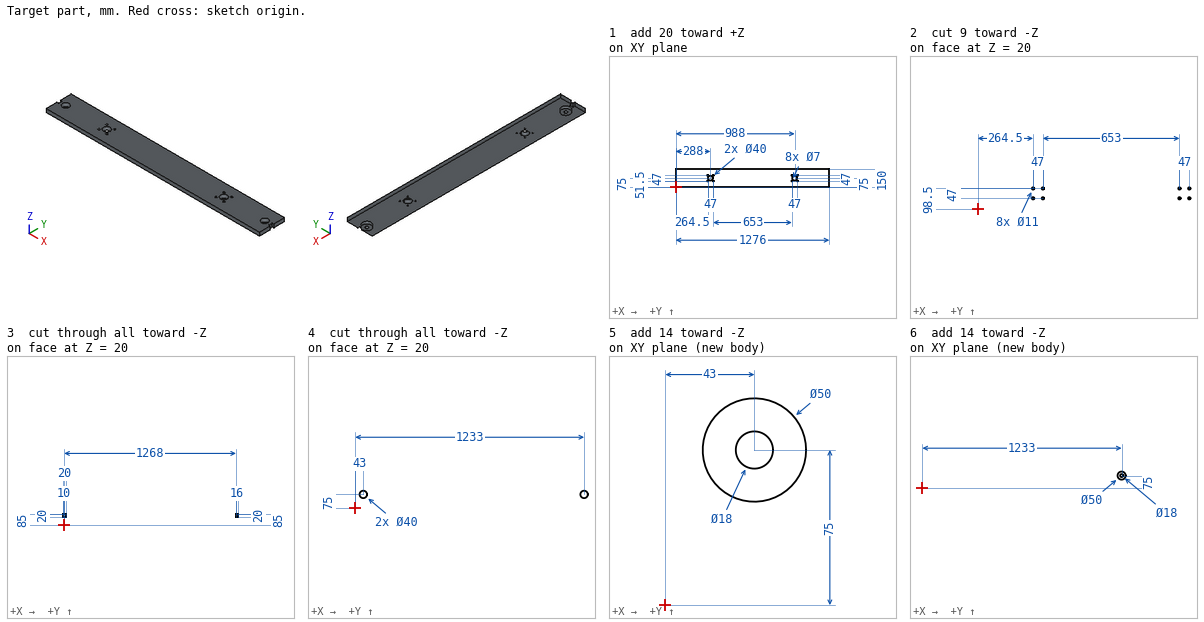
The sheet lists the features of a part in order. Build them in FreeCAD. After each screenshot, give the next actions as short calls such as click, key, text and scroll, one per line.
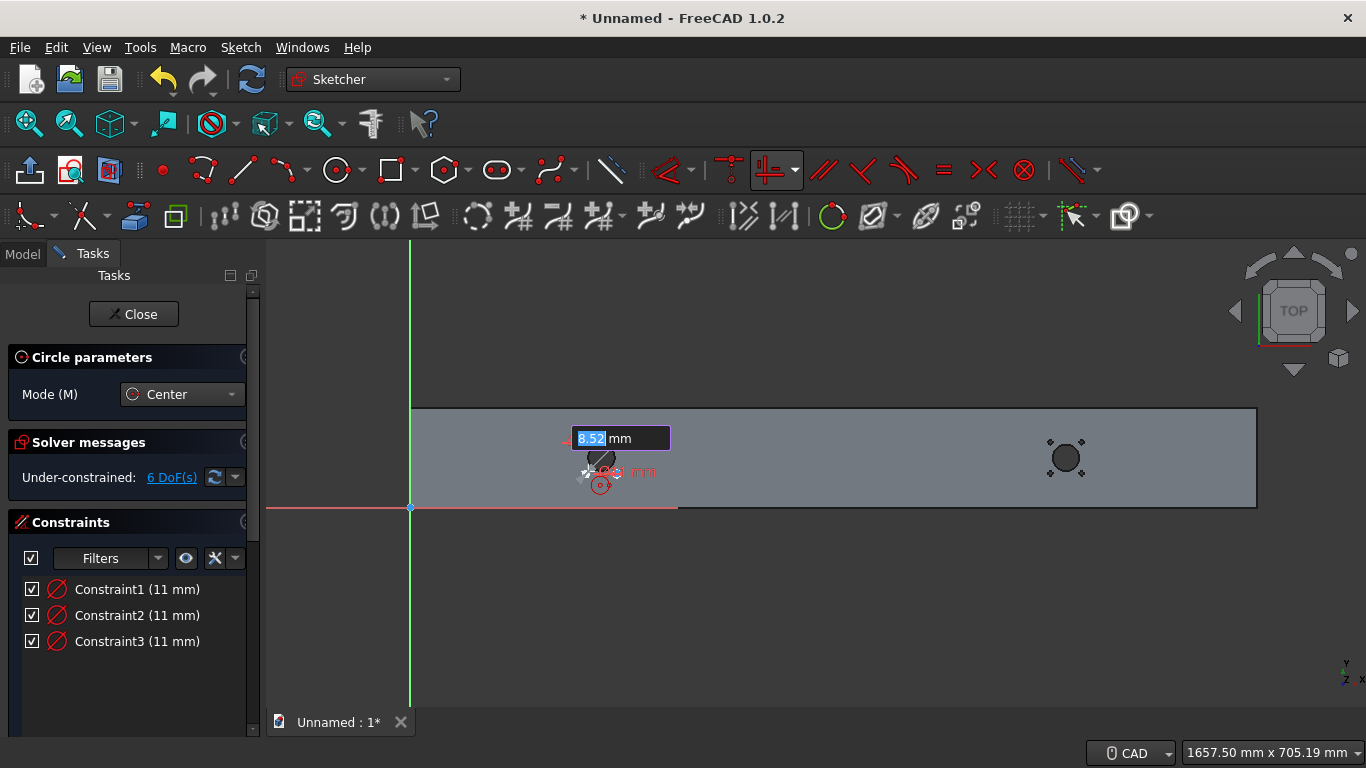
text(11)
key(Return)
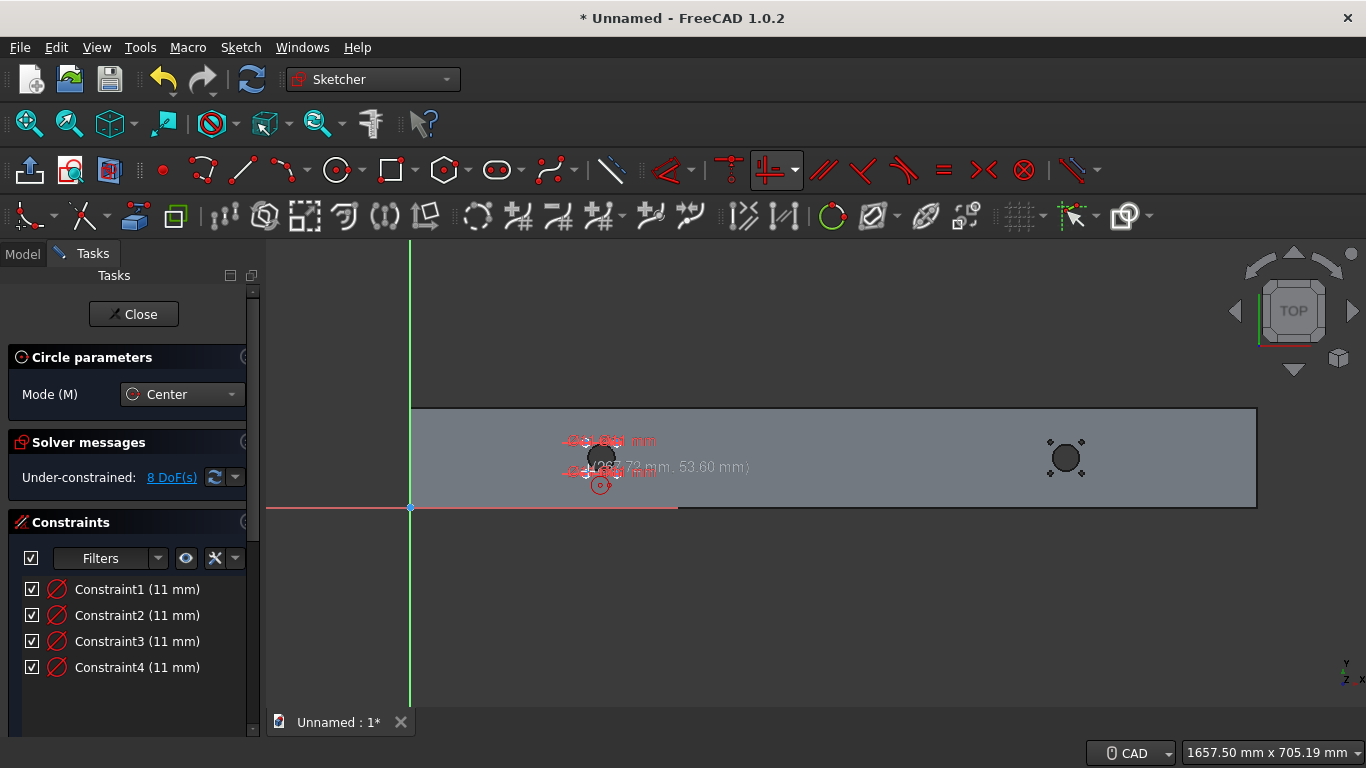
scroll(1050, 442, up, 10)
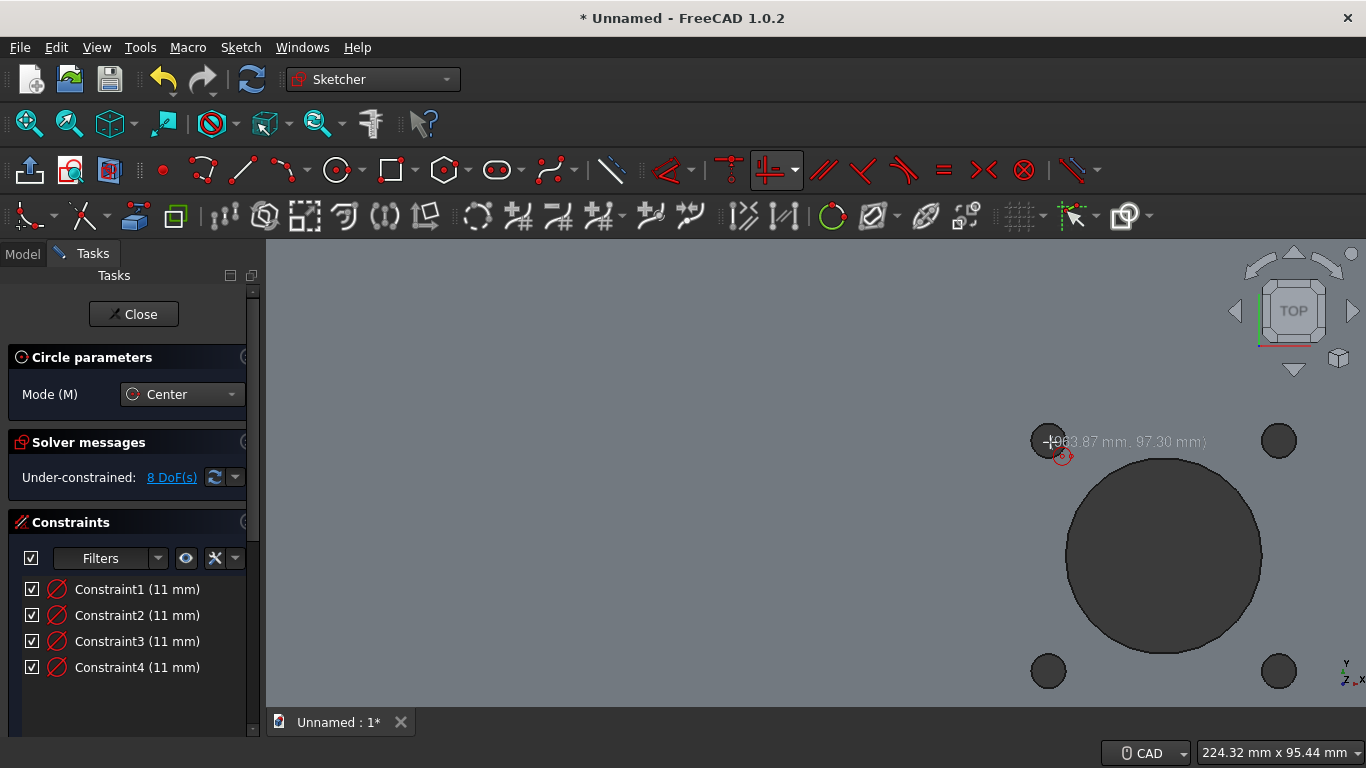
scroll(1050, 442, down, 10)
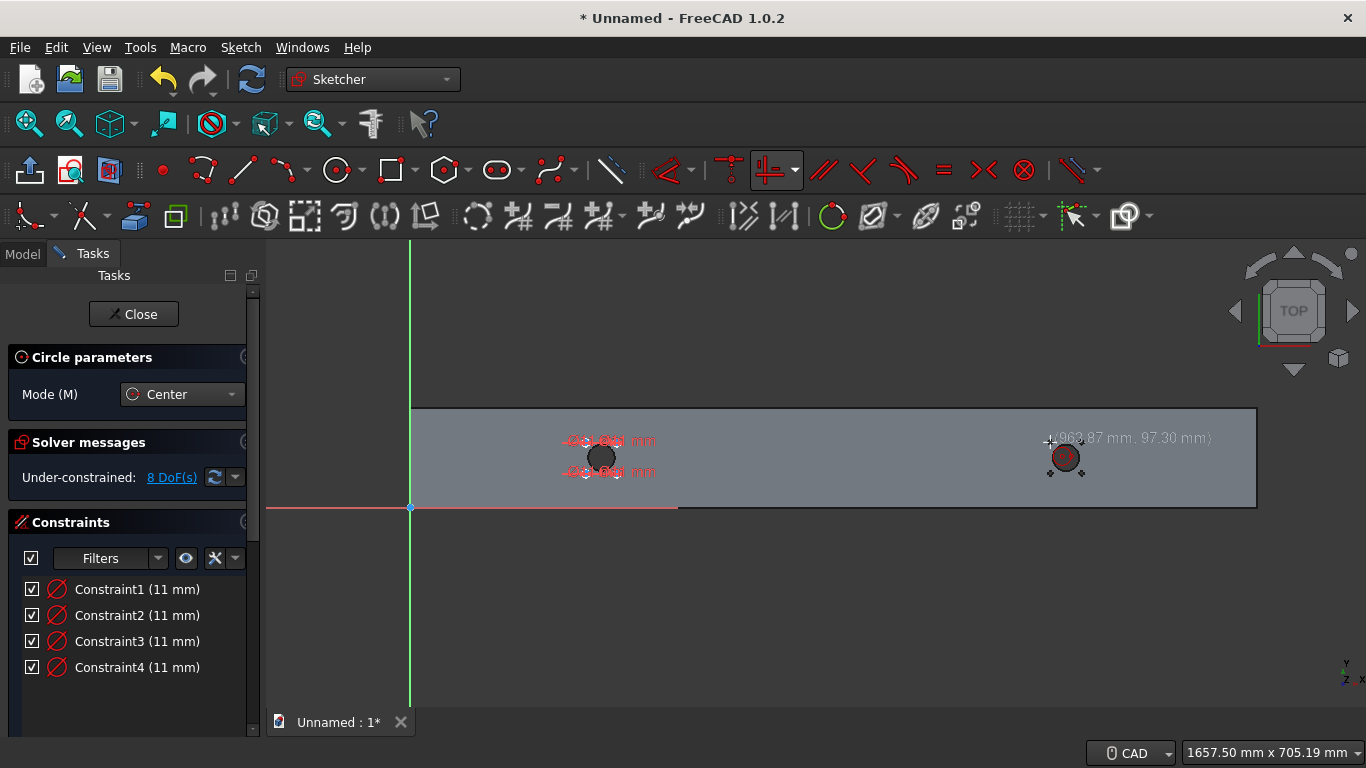
click(1050, 442)
move(1053, 440)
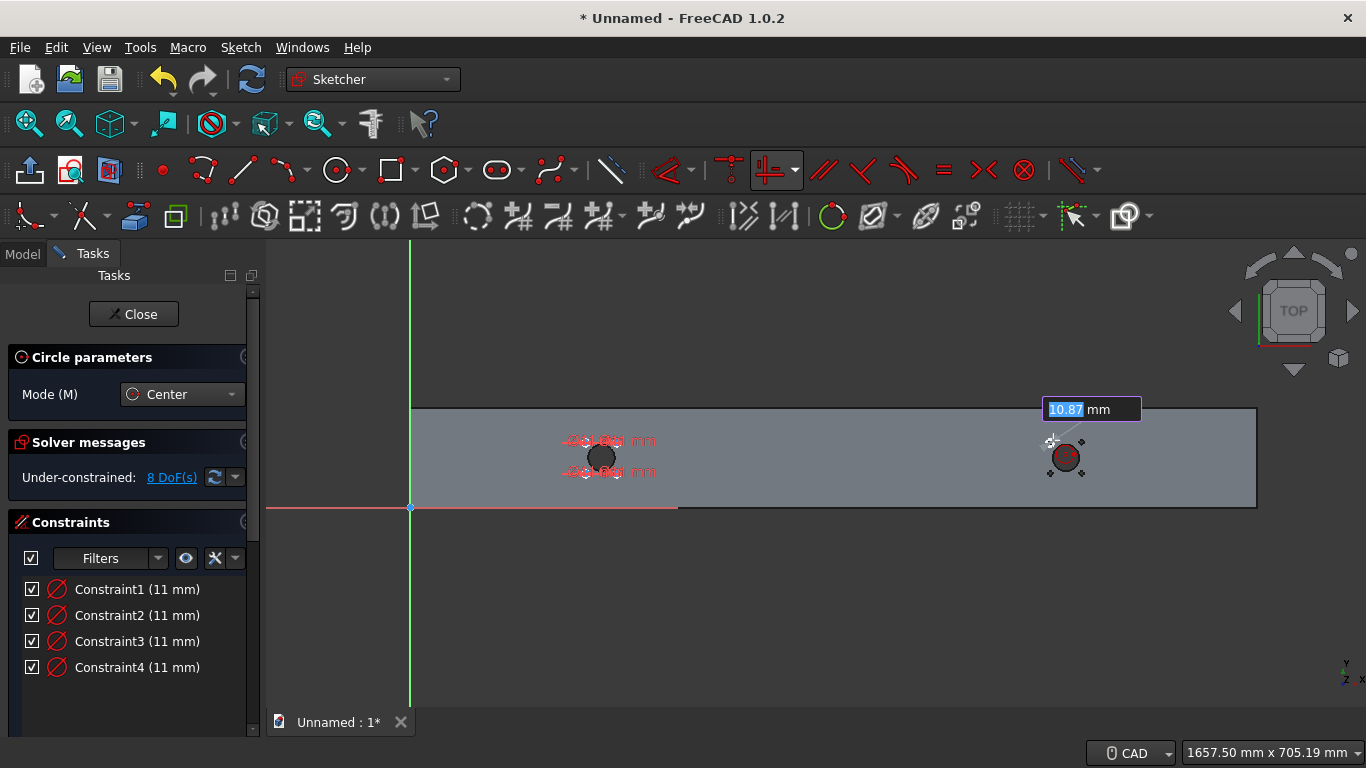
text(11)
key(Return)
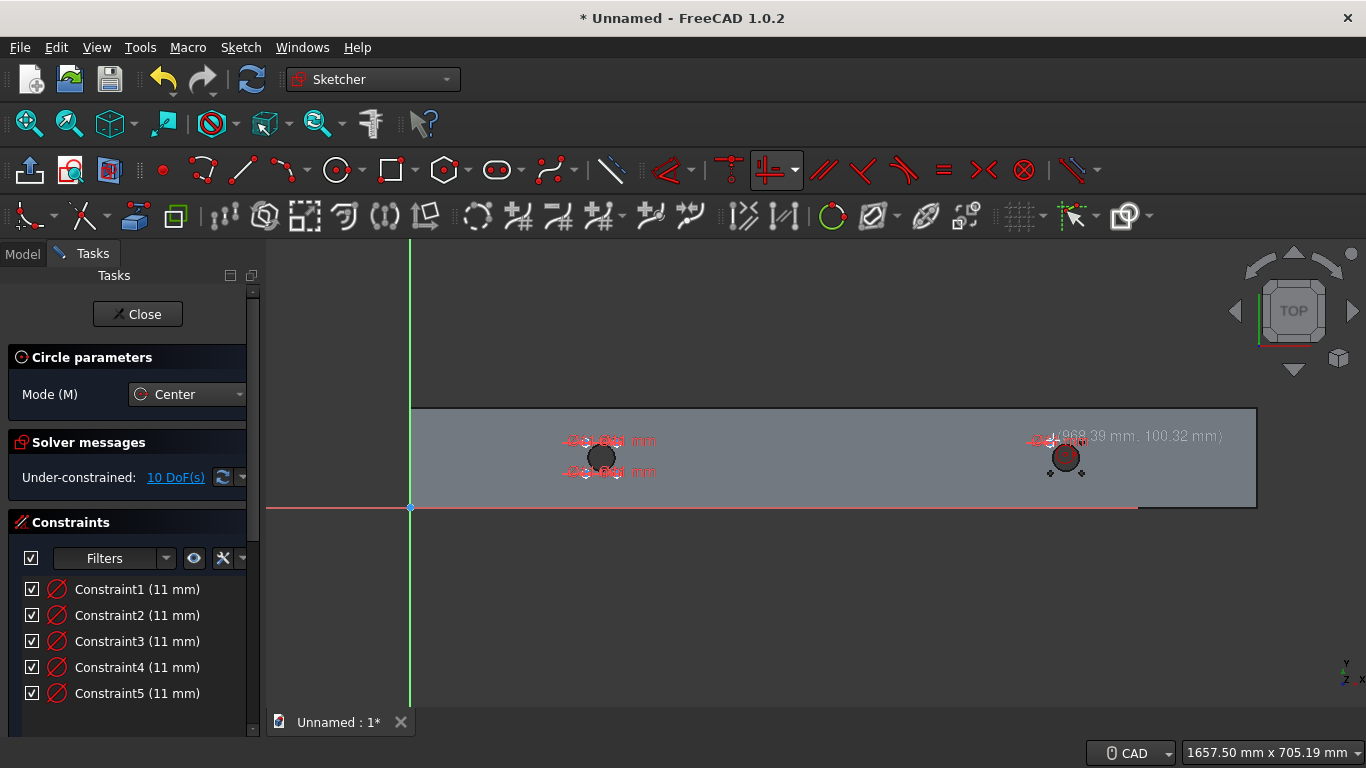
scroll(1082, 442, up, 10)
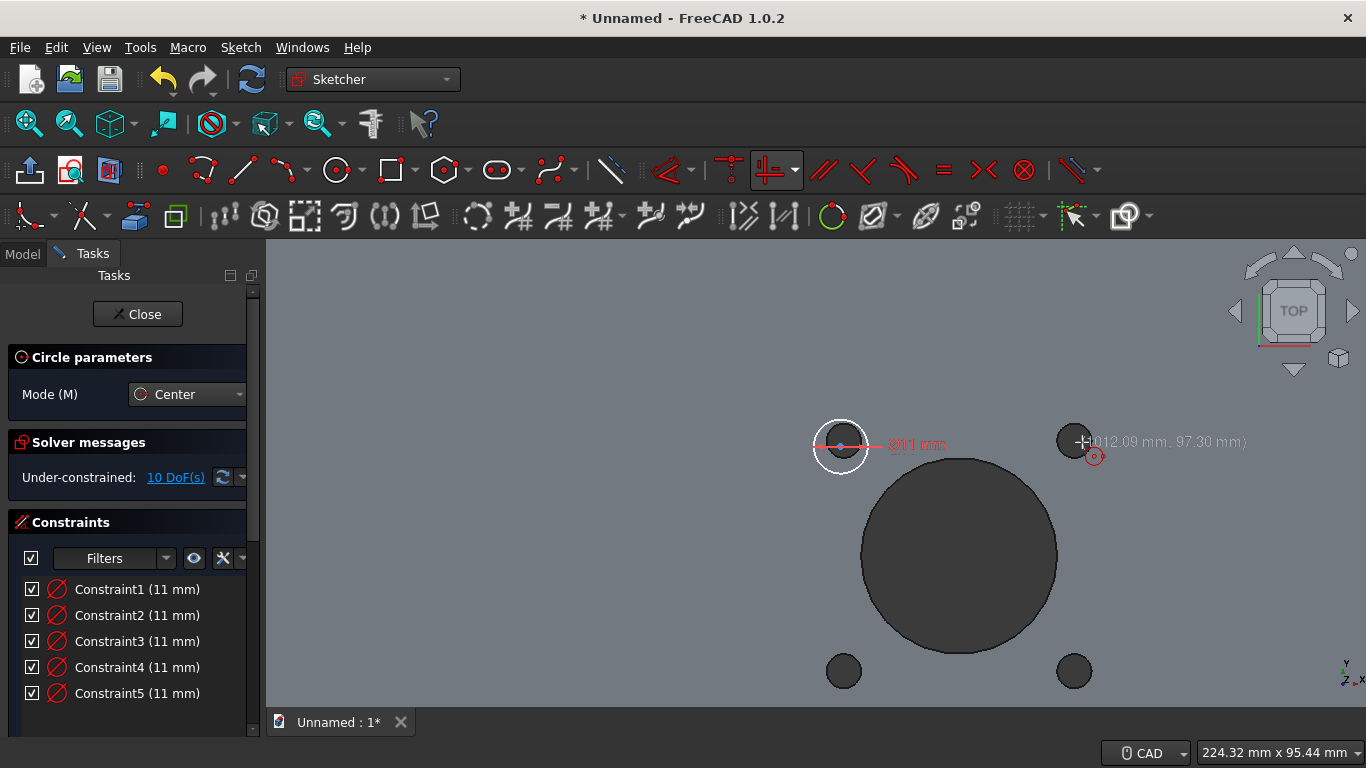
scroll(1082, 442, down, 10)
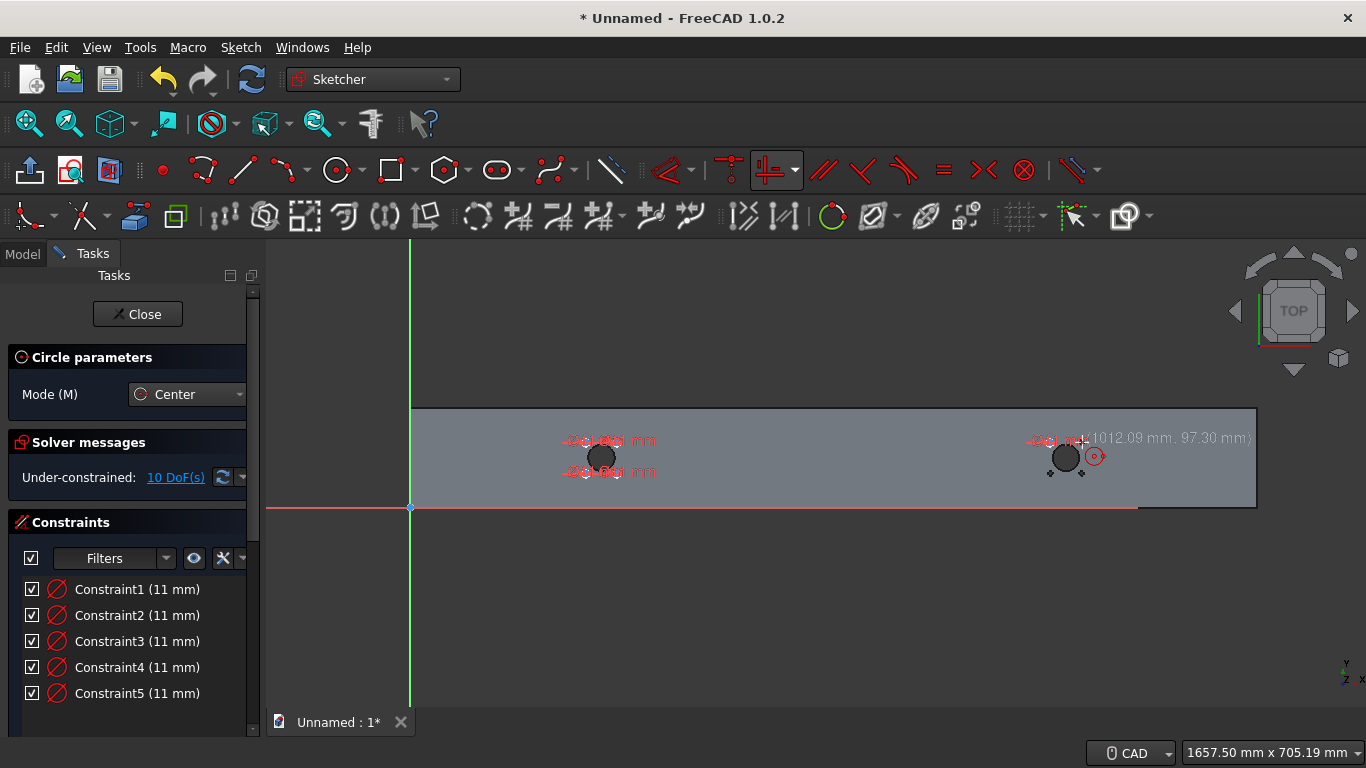
click(1082, 442)
move(1084, 440)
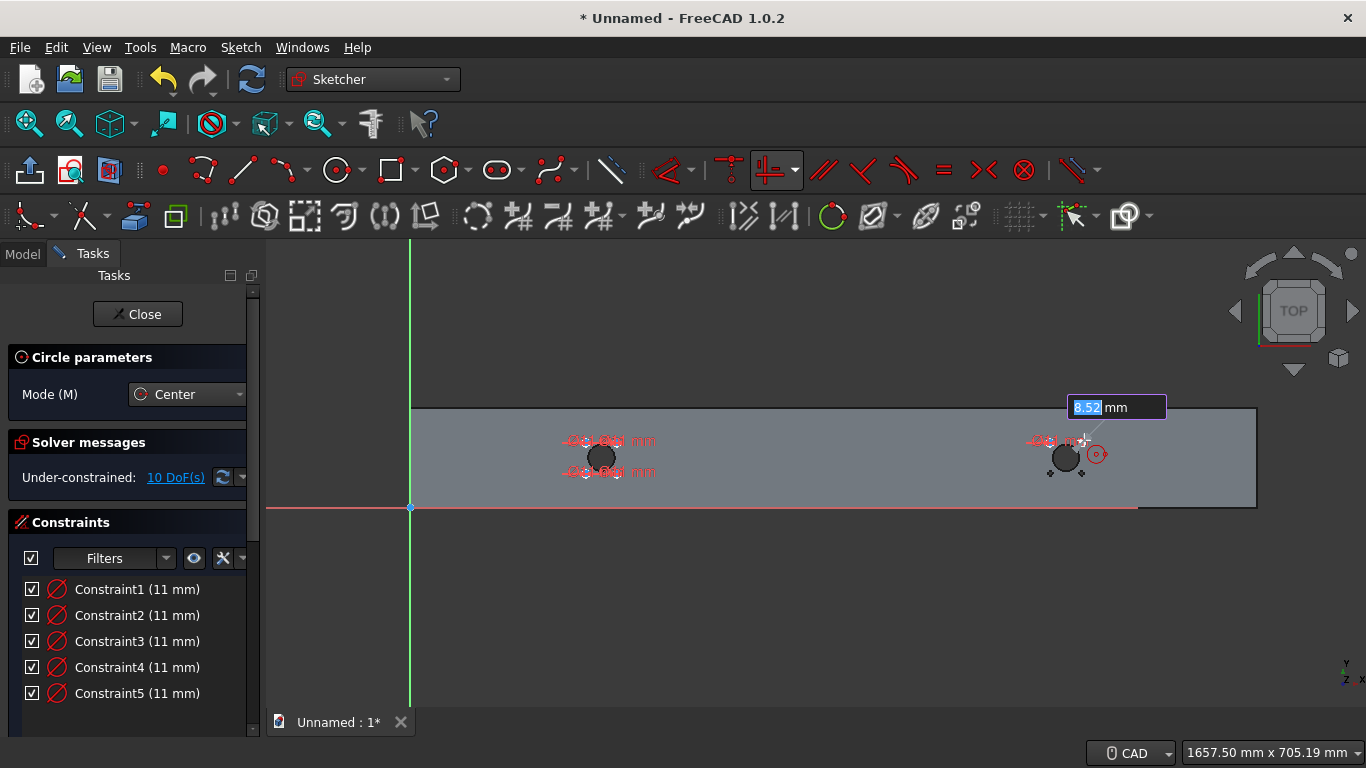
text(11)
key(Return)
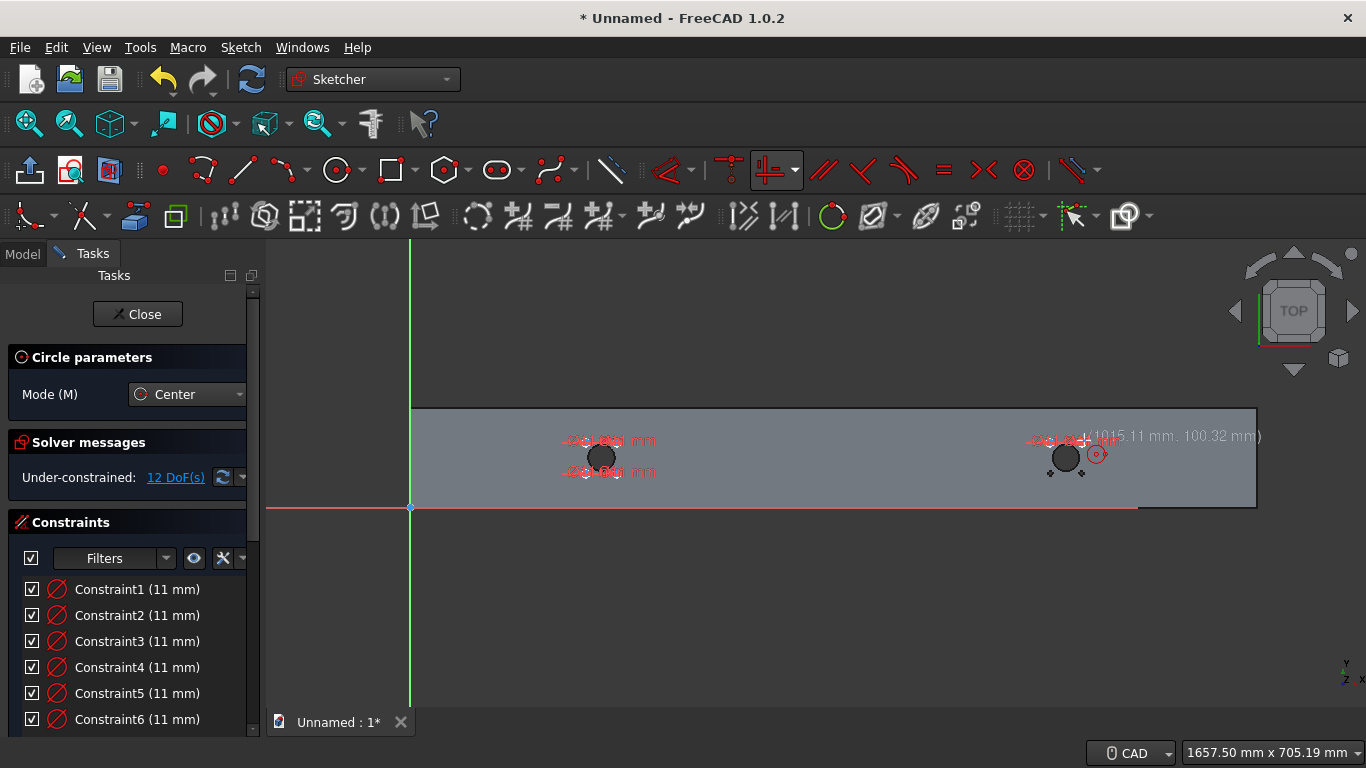
scroll(1082, 473, up, 10)